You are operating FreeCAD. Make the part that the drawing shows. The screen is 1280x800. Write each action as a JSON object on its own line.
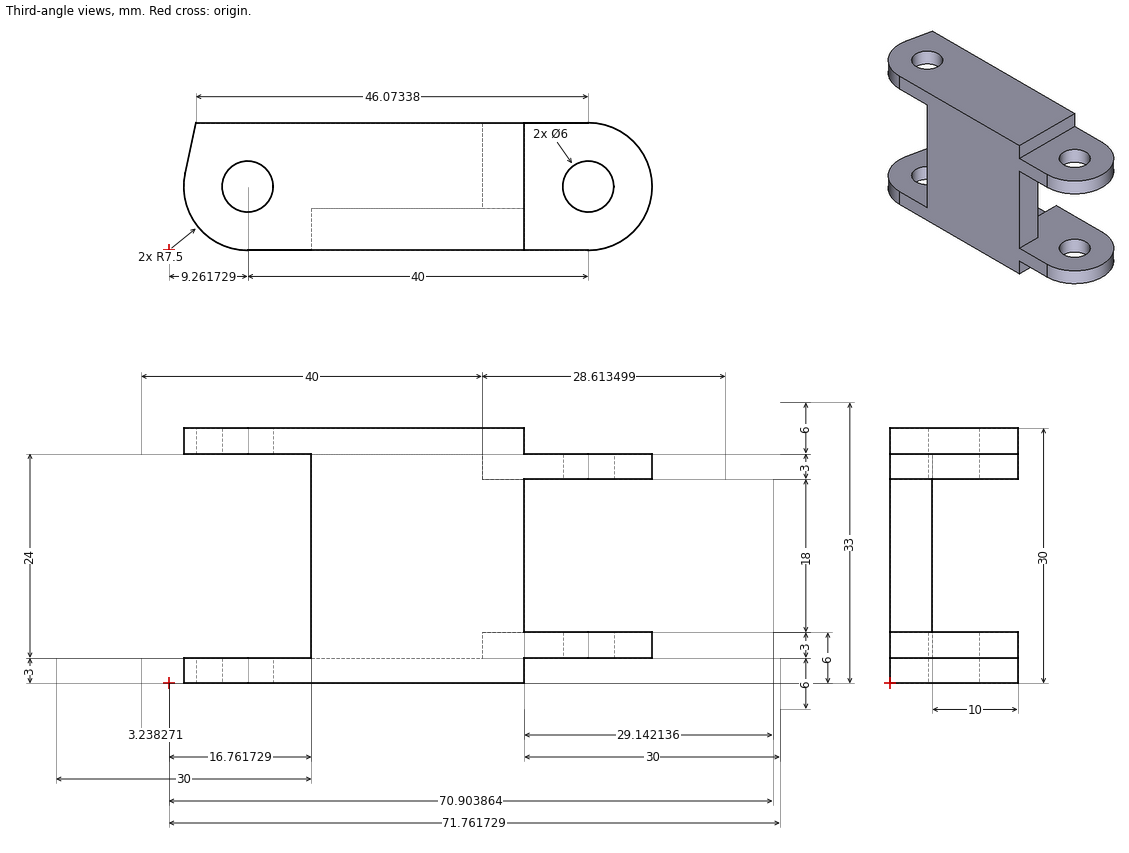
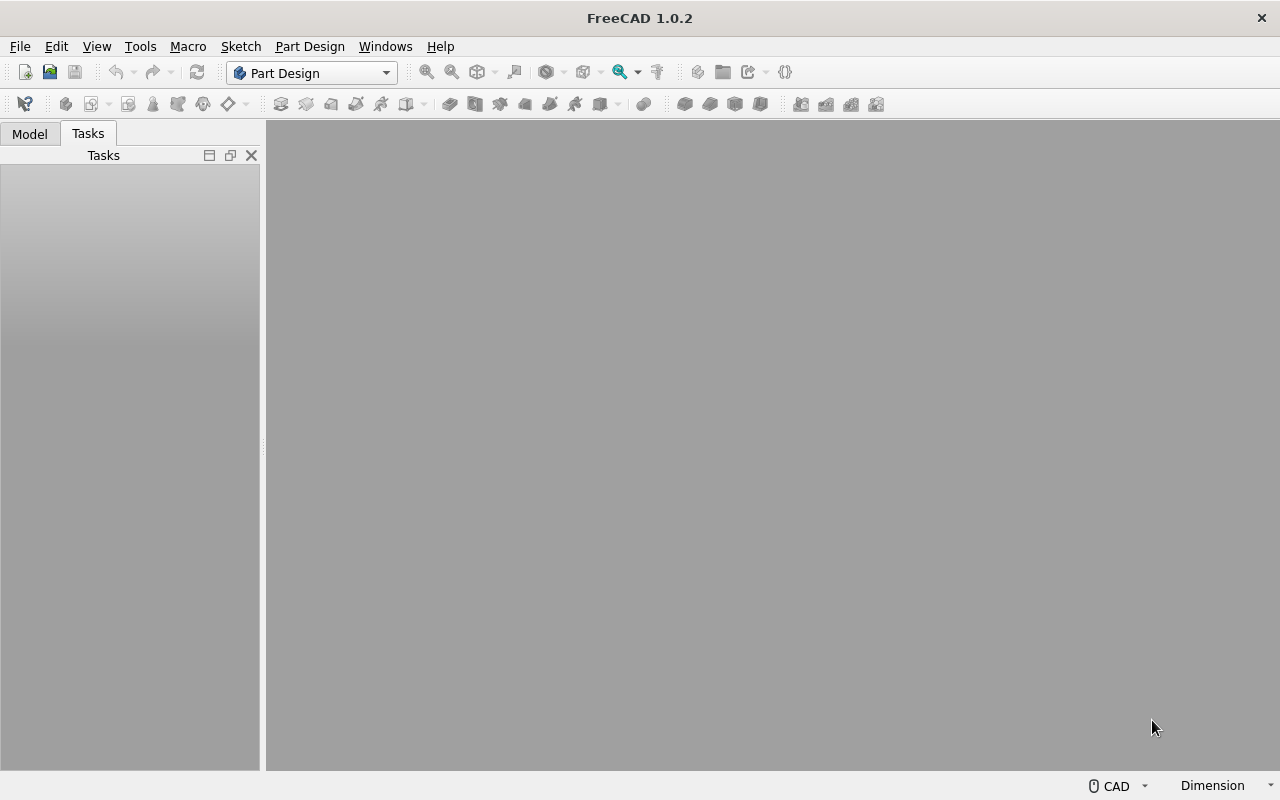
{"action": "left_click", "coordinate": [25, 72]}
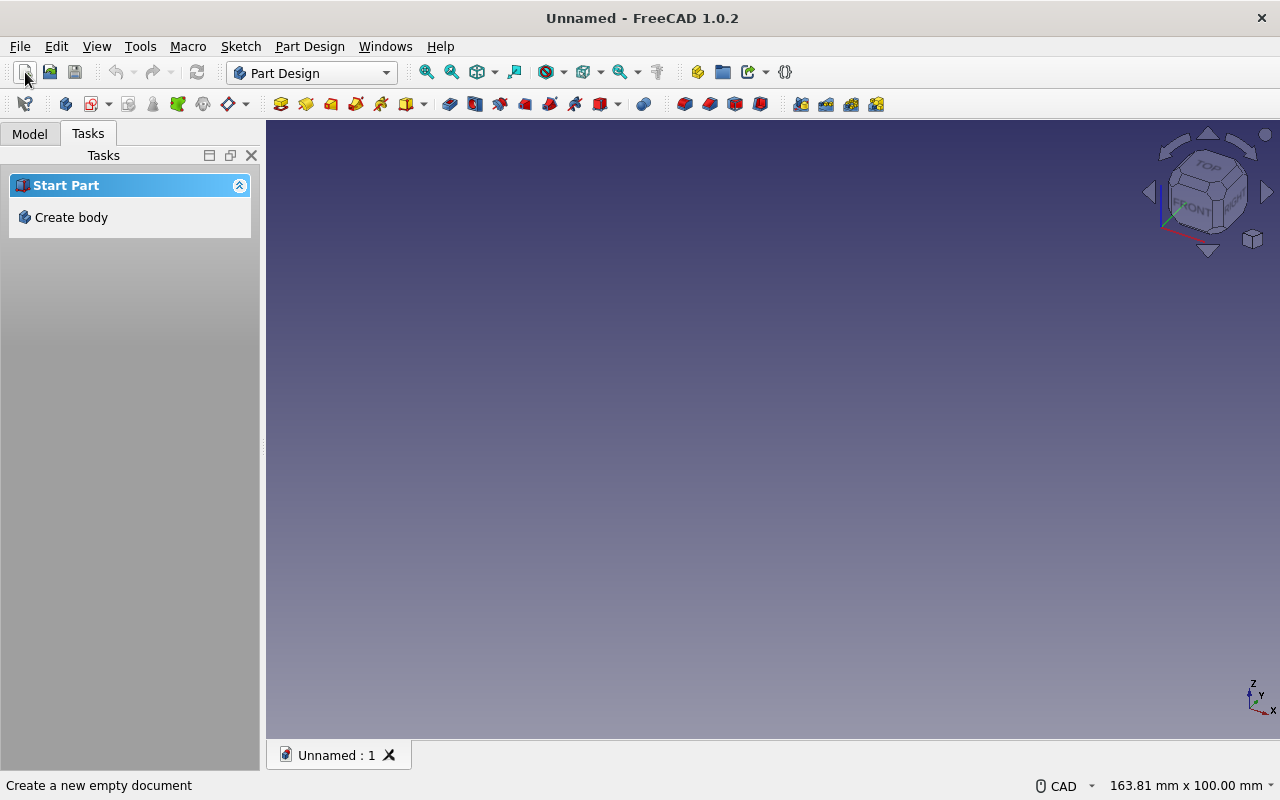
{"action": "left_click", "coordinate": [90, 104]}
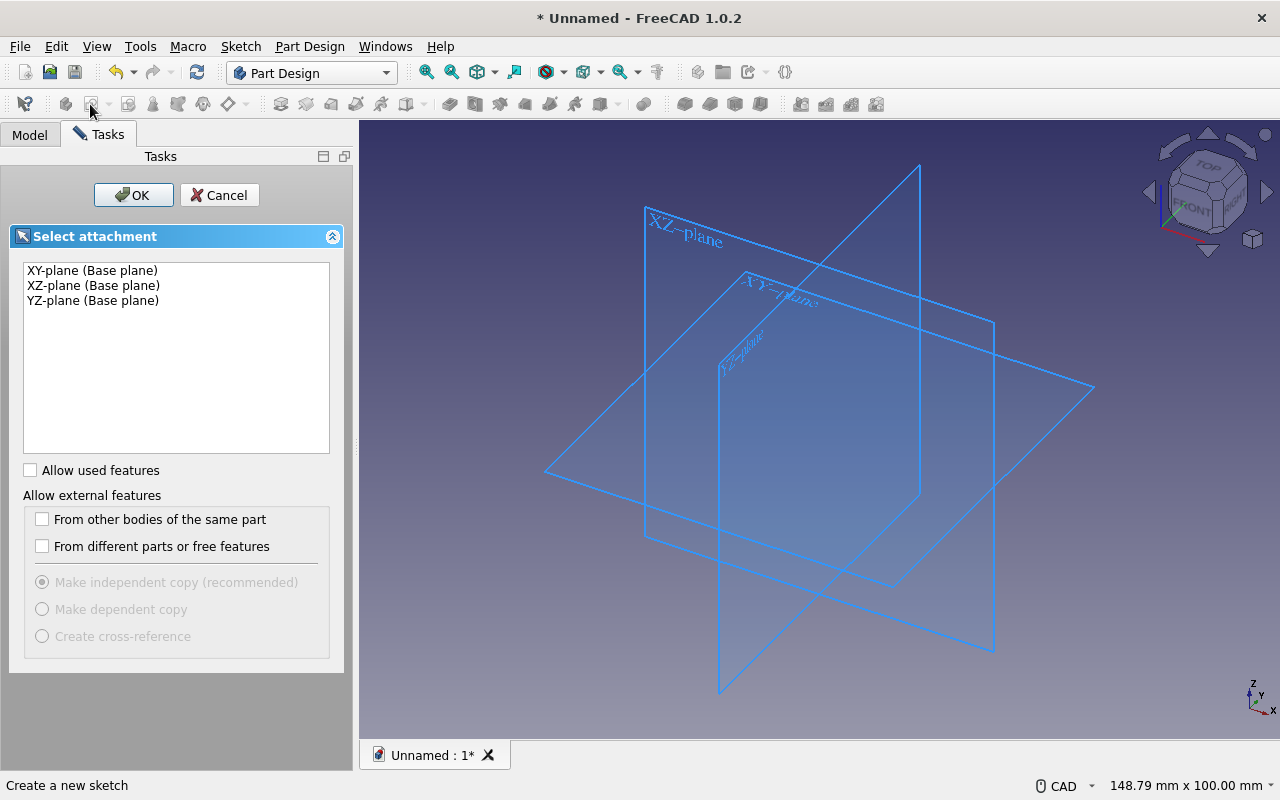
{"action": "left_click", "coordinate": [84, 270]}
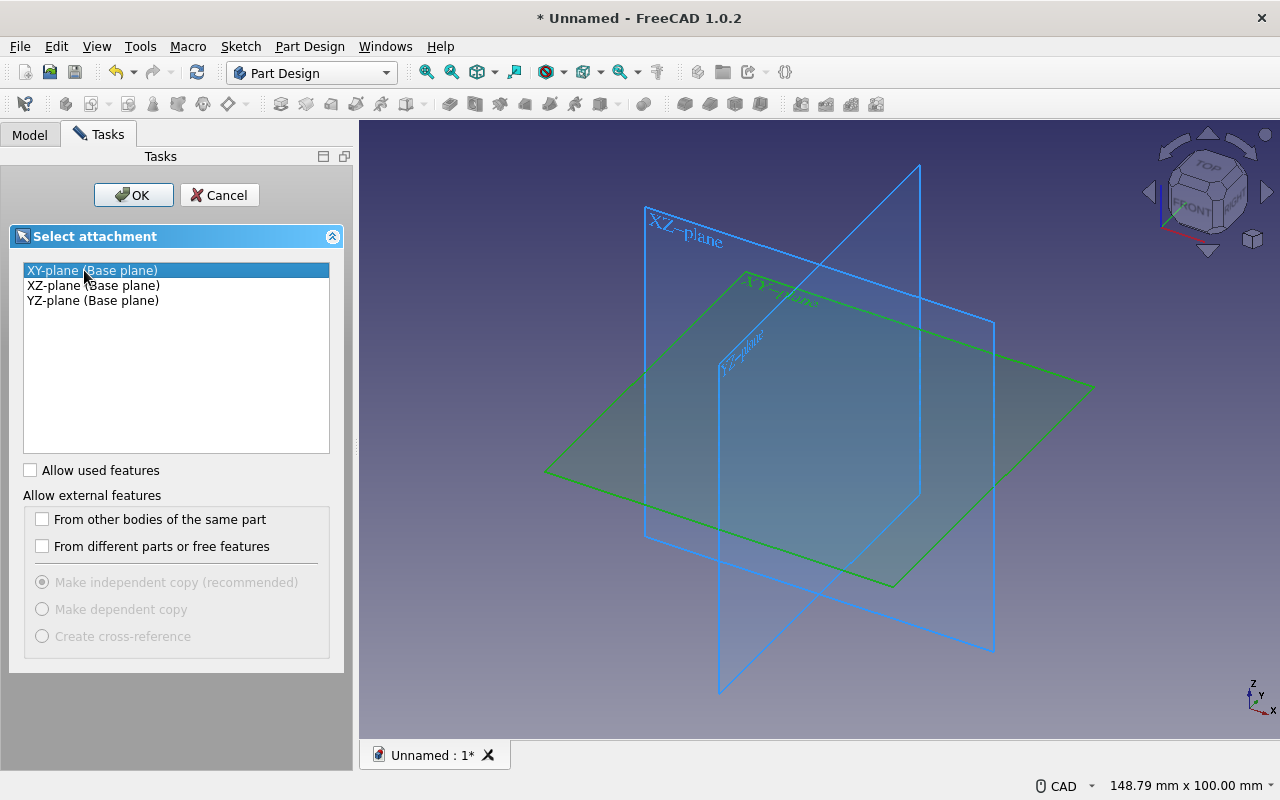
{"action": "left_click", "coordinate": [134, 195]}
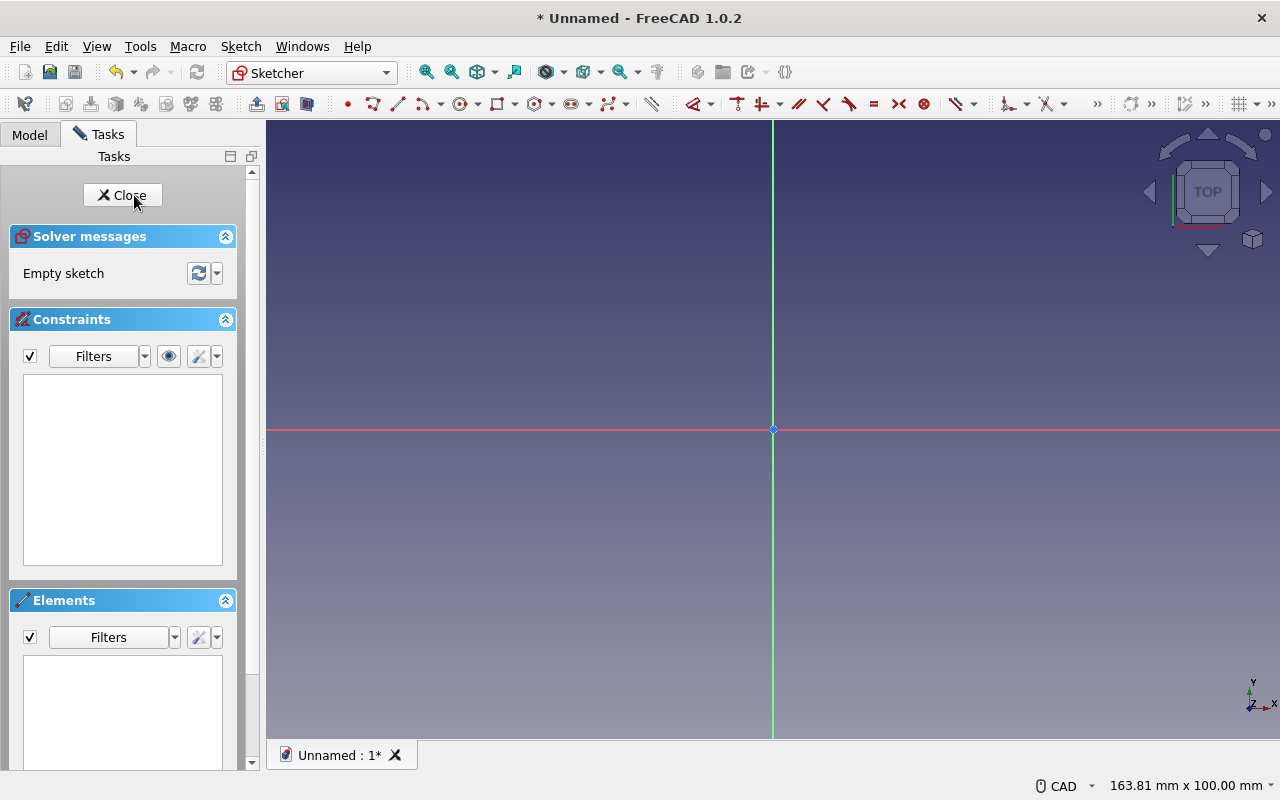
{"action": "scroll", "coordinate": [704, 430], "scroll_direction": "down", "scroll_amount": 5}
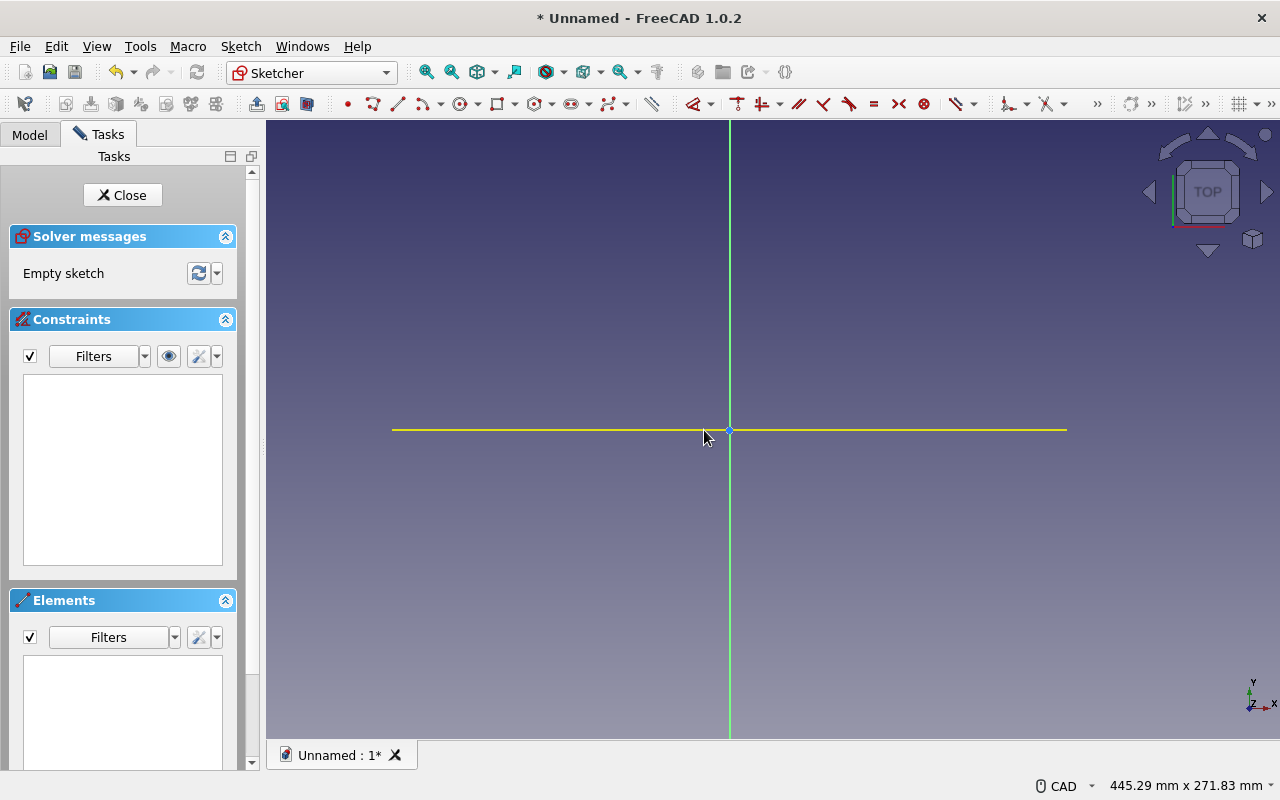
{"action": "scroll", "coordinate": [817, 409], "scroll_direction": "up", "scroll_amount": 8}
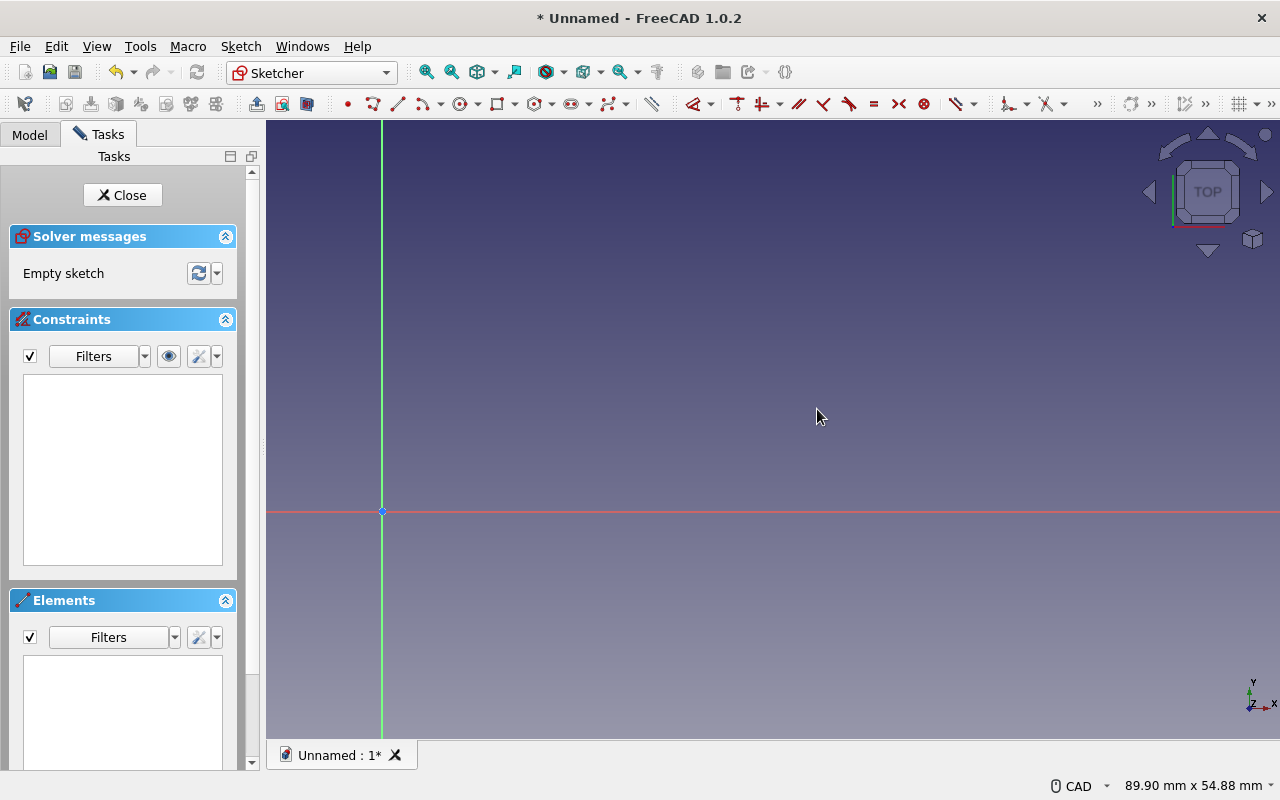
{"action": "left_click", "coordinate": [398, 104]}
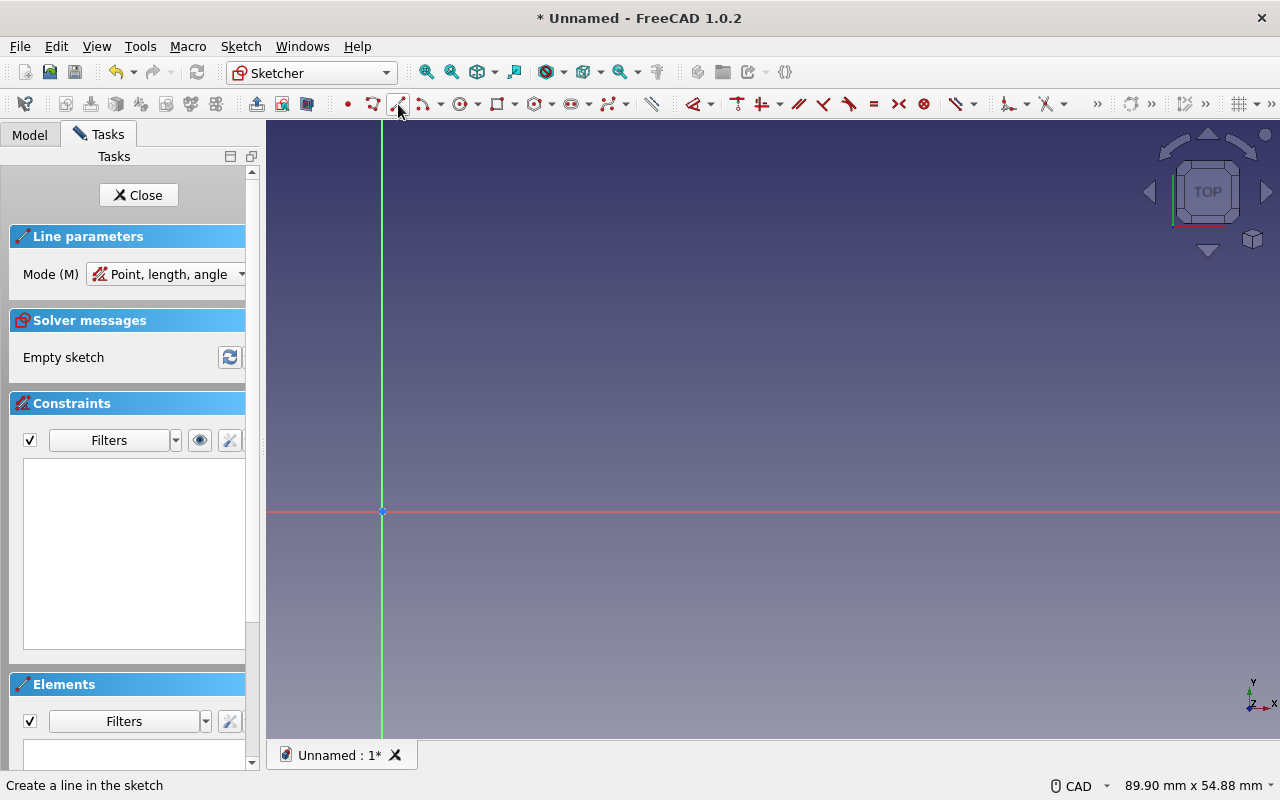
{"action": "left_click", "coordinate": [487, 512]}
{"action": "left_click", "coordinate": [938, 503]}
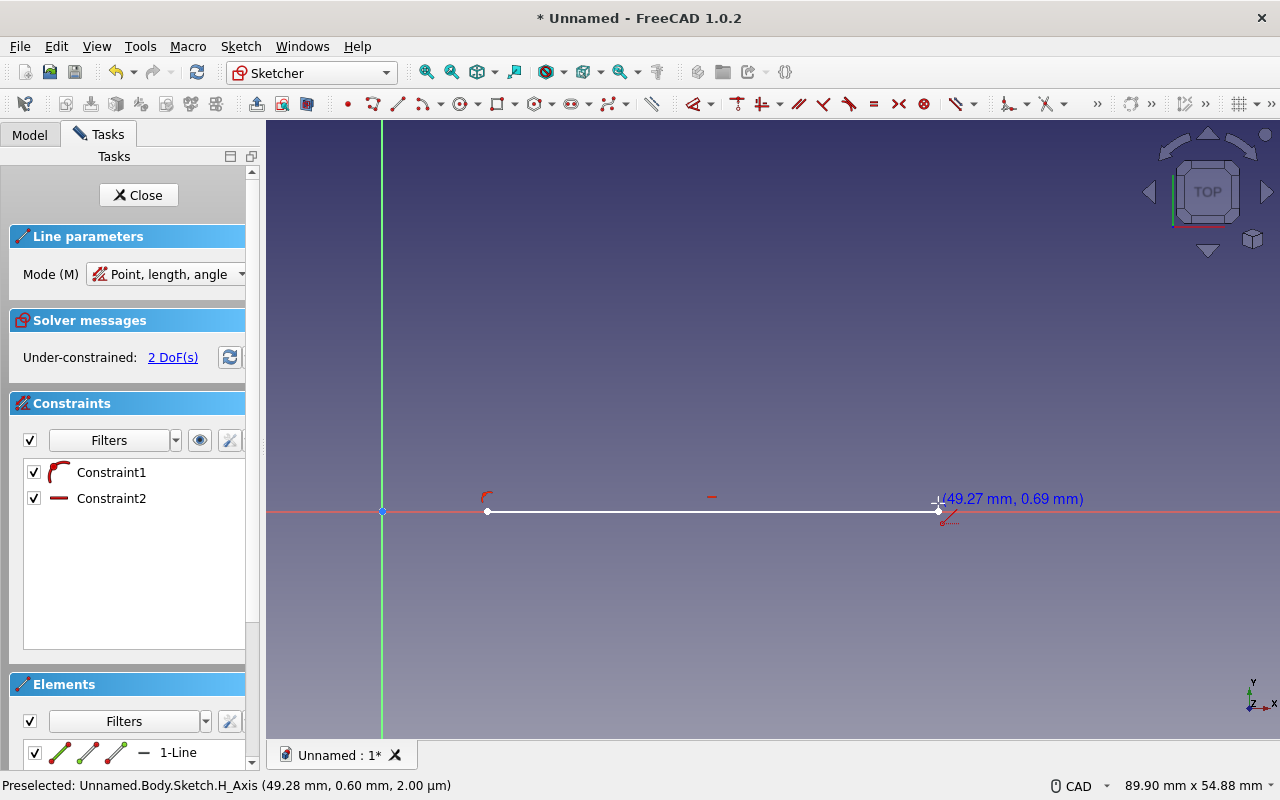
{"action": "left_click", "coordinate": [373, 104]}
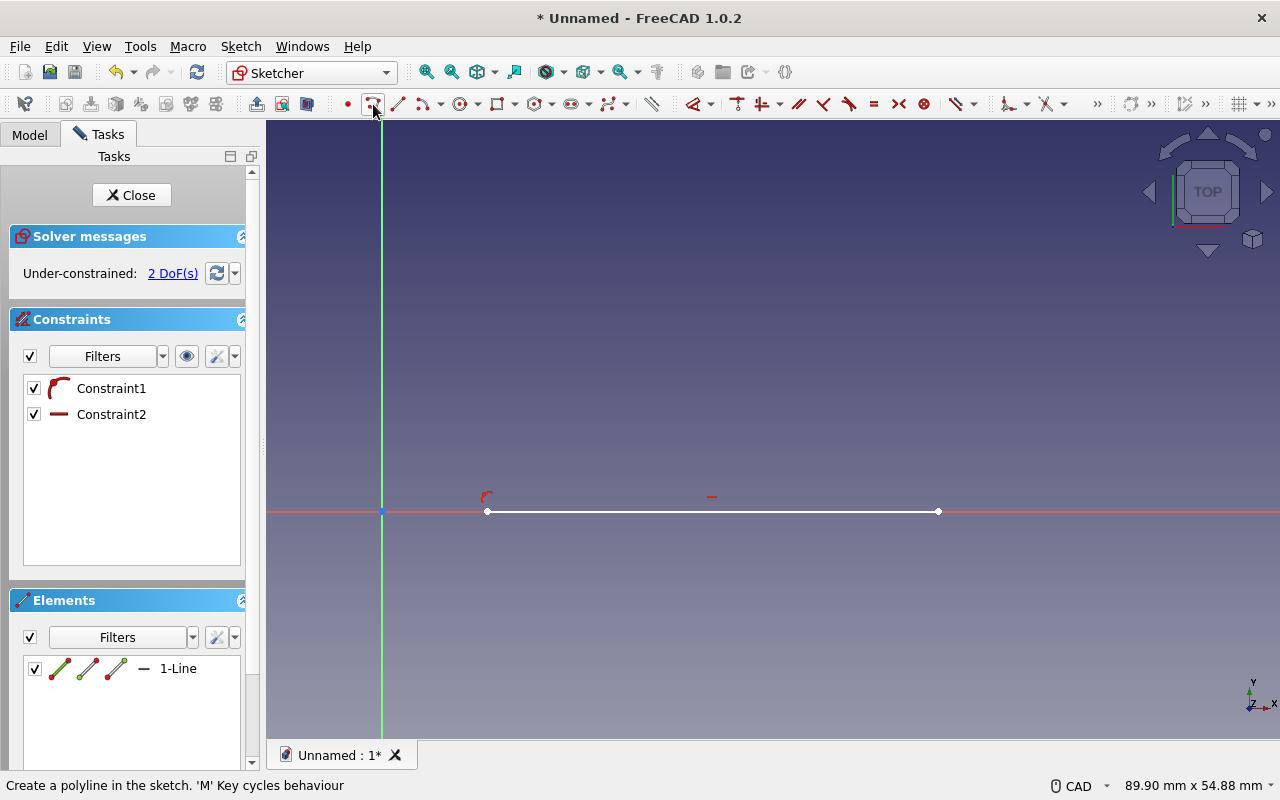
{"action": "left_click", "coordinate": [938, 343]}
{"action": "left_click", "coordinate": [418, 343]}
{"action": "left_click", "coordinate": [404, 410]}
{"action": "right_click", "coordinate": [404, 410]}